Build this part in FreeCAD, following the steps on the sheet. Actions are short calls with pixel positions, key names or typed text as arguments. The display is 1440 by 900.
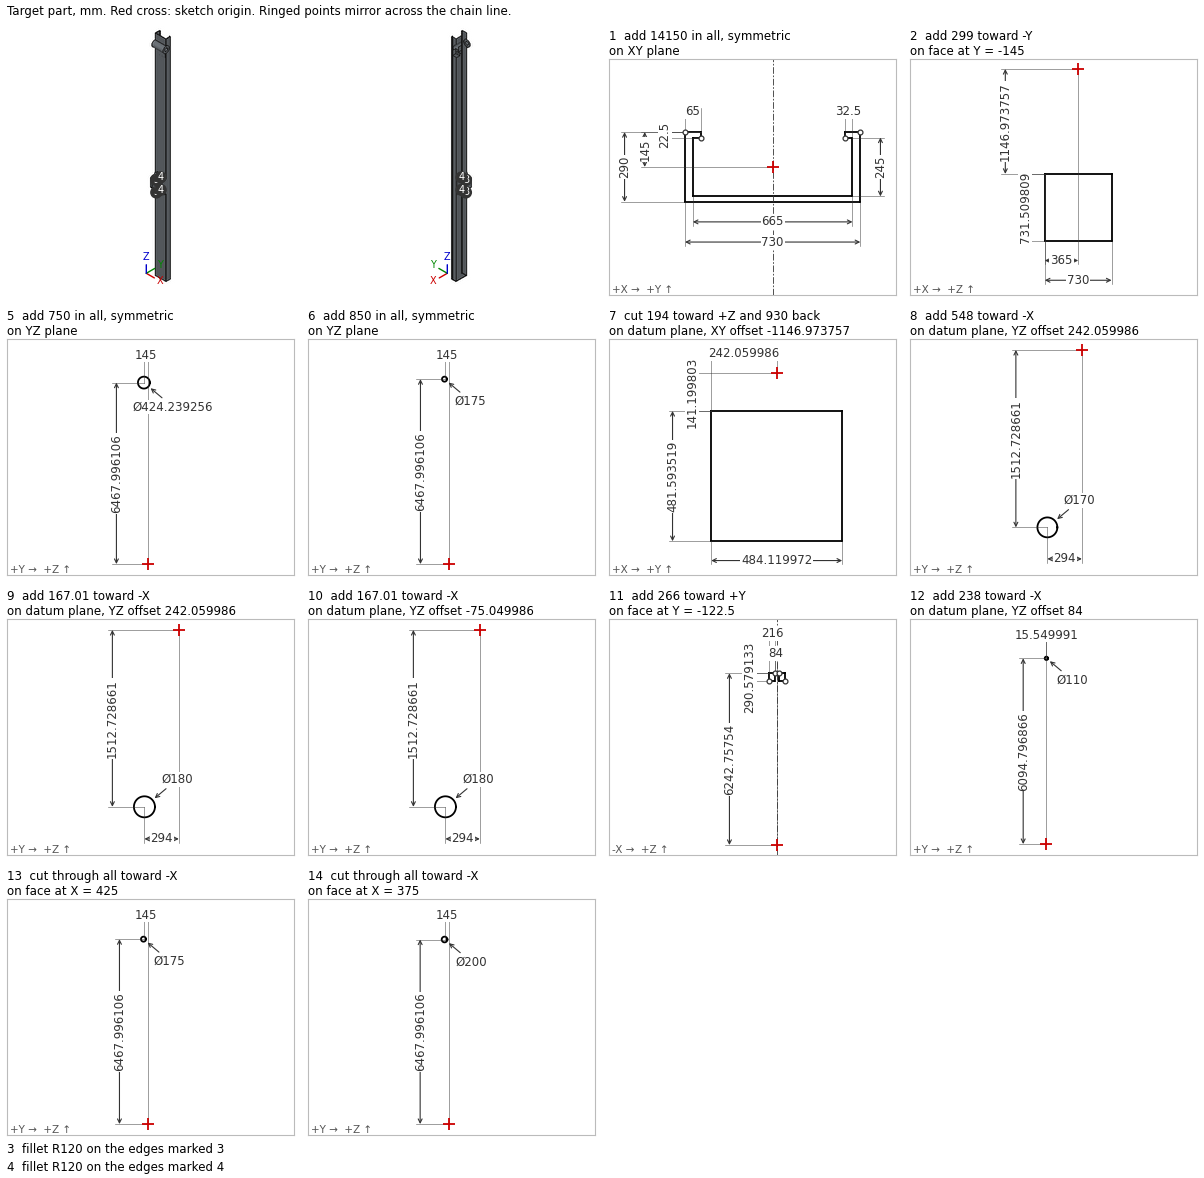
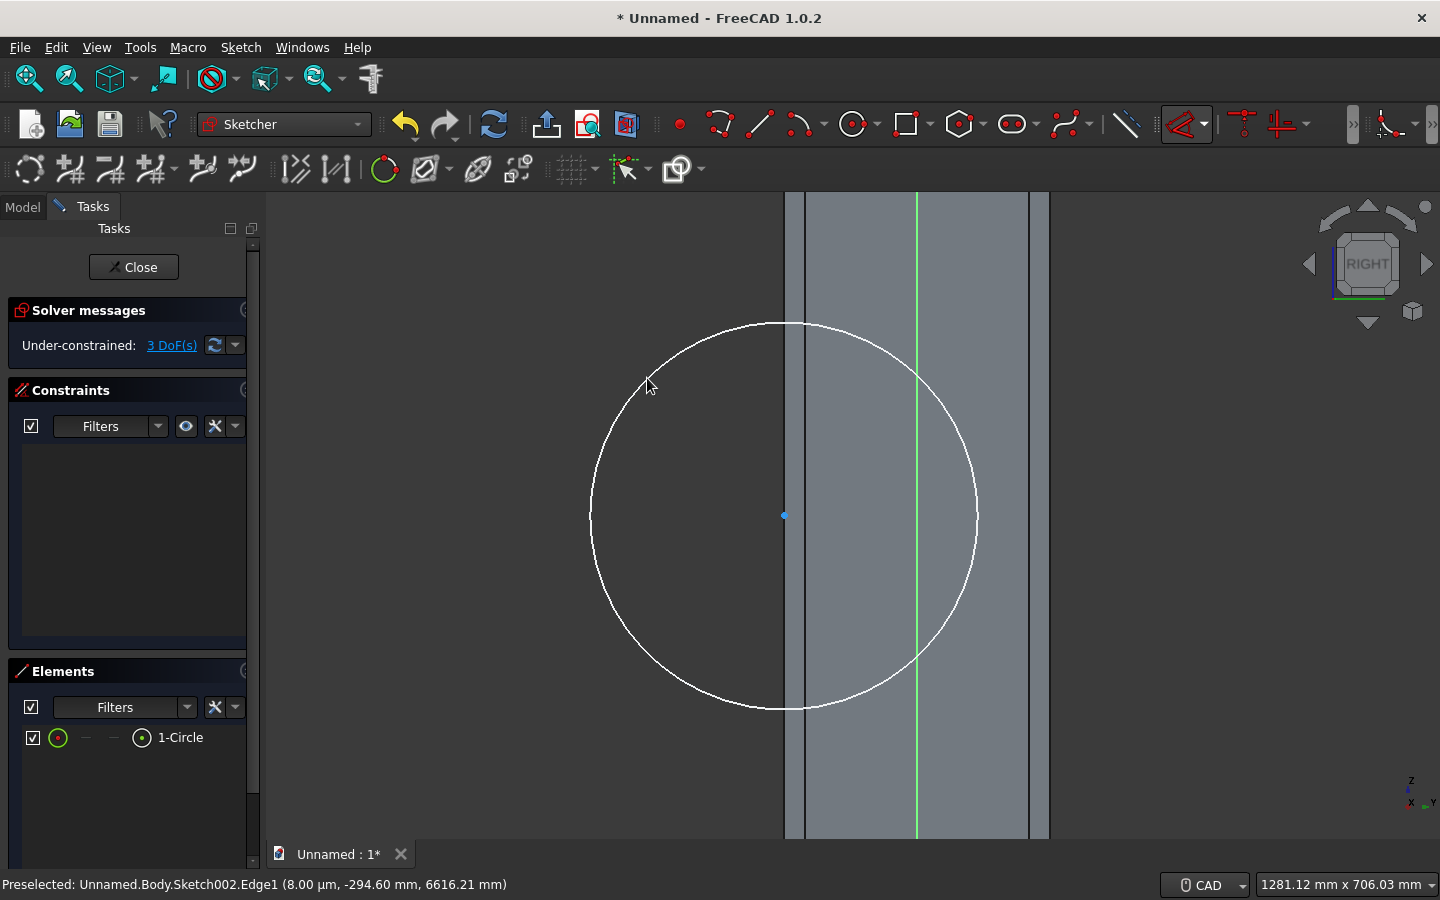
click(921, 379)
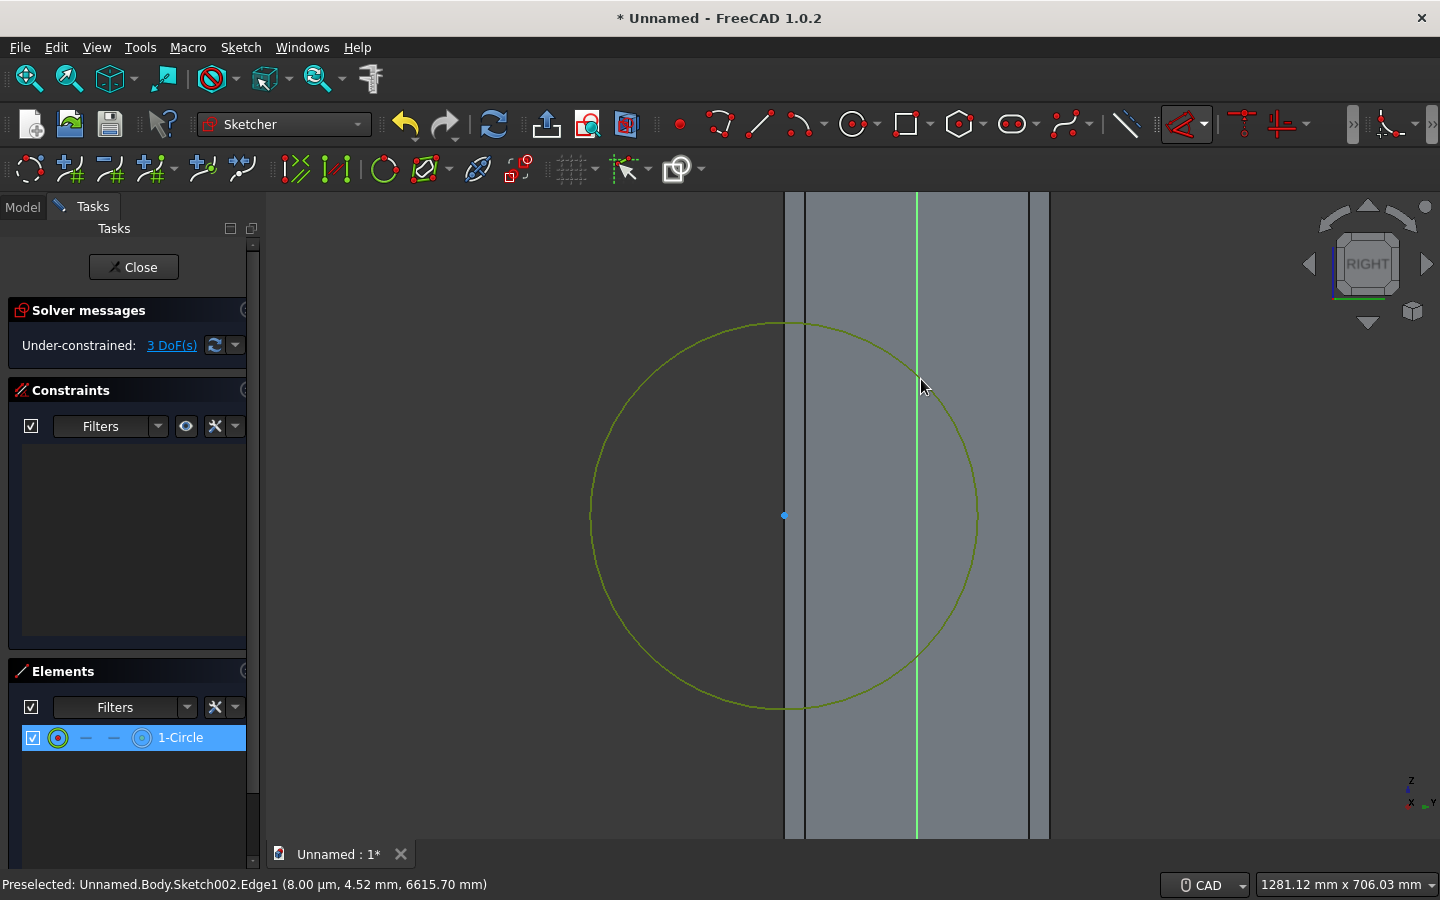
key(k)
key(o)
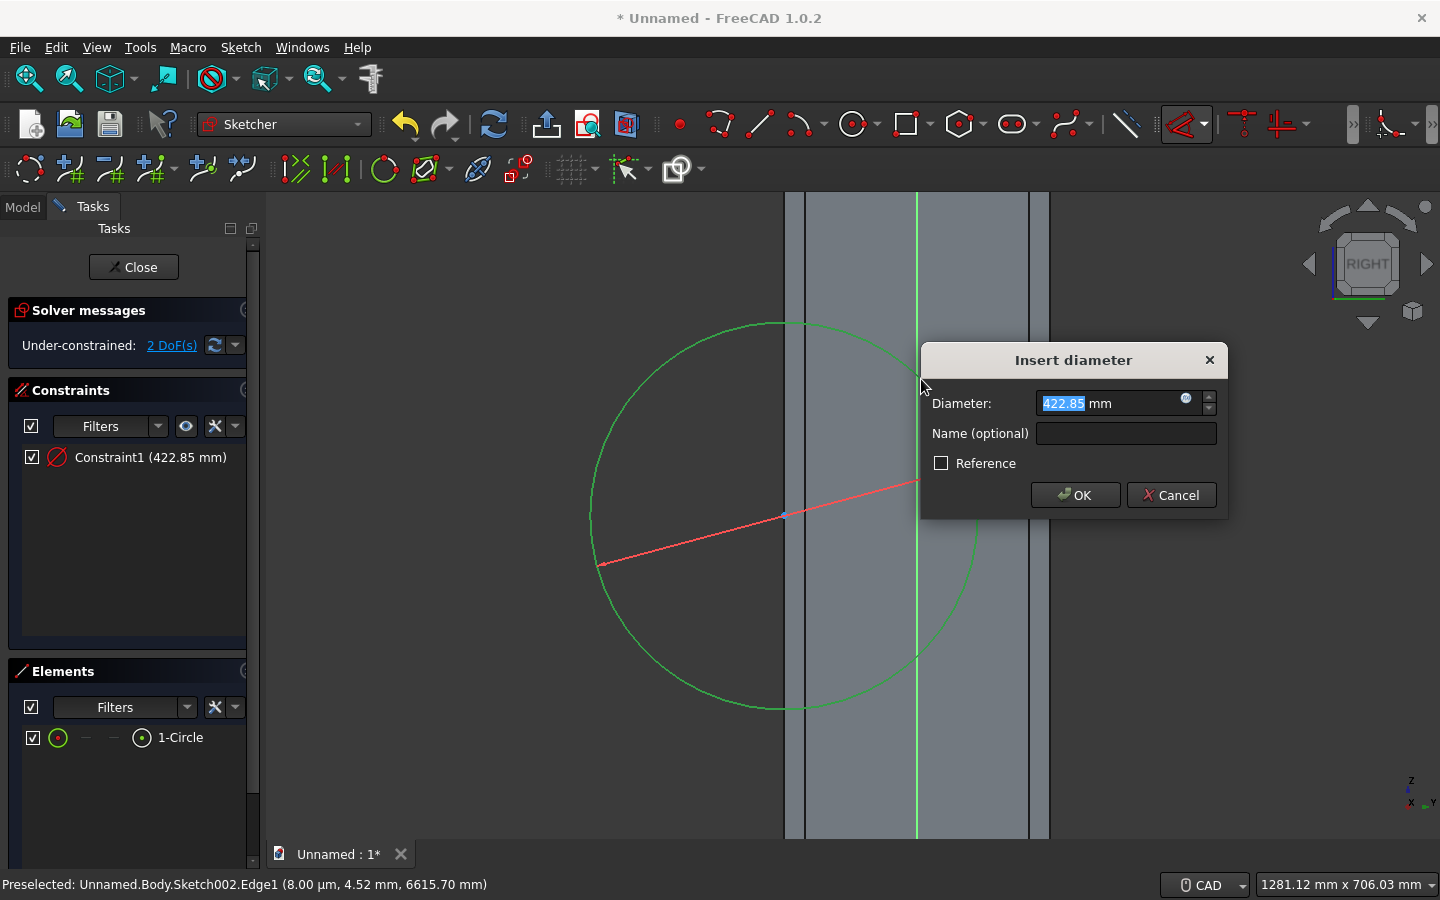
text(424.239256)
key(Return)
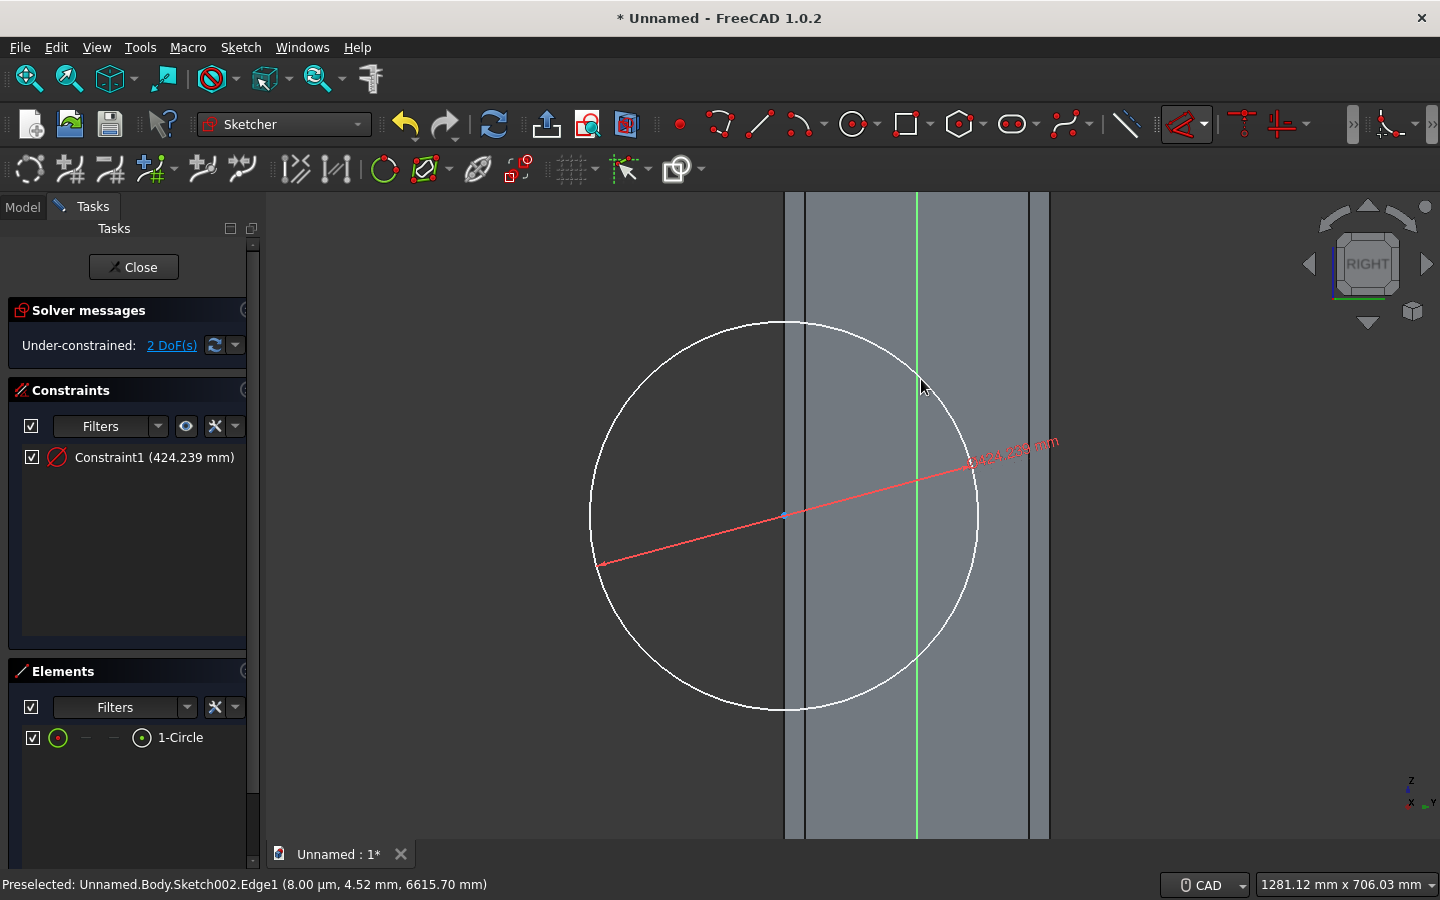
click(784, 516)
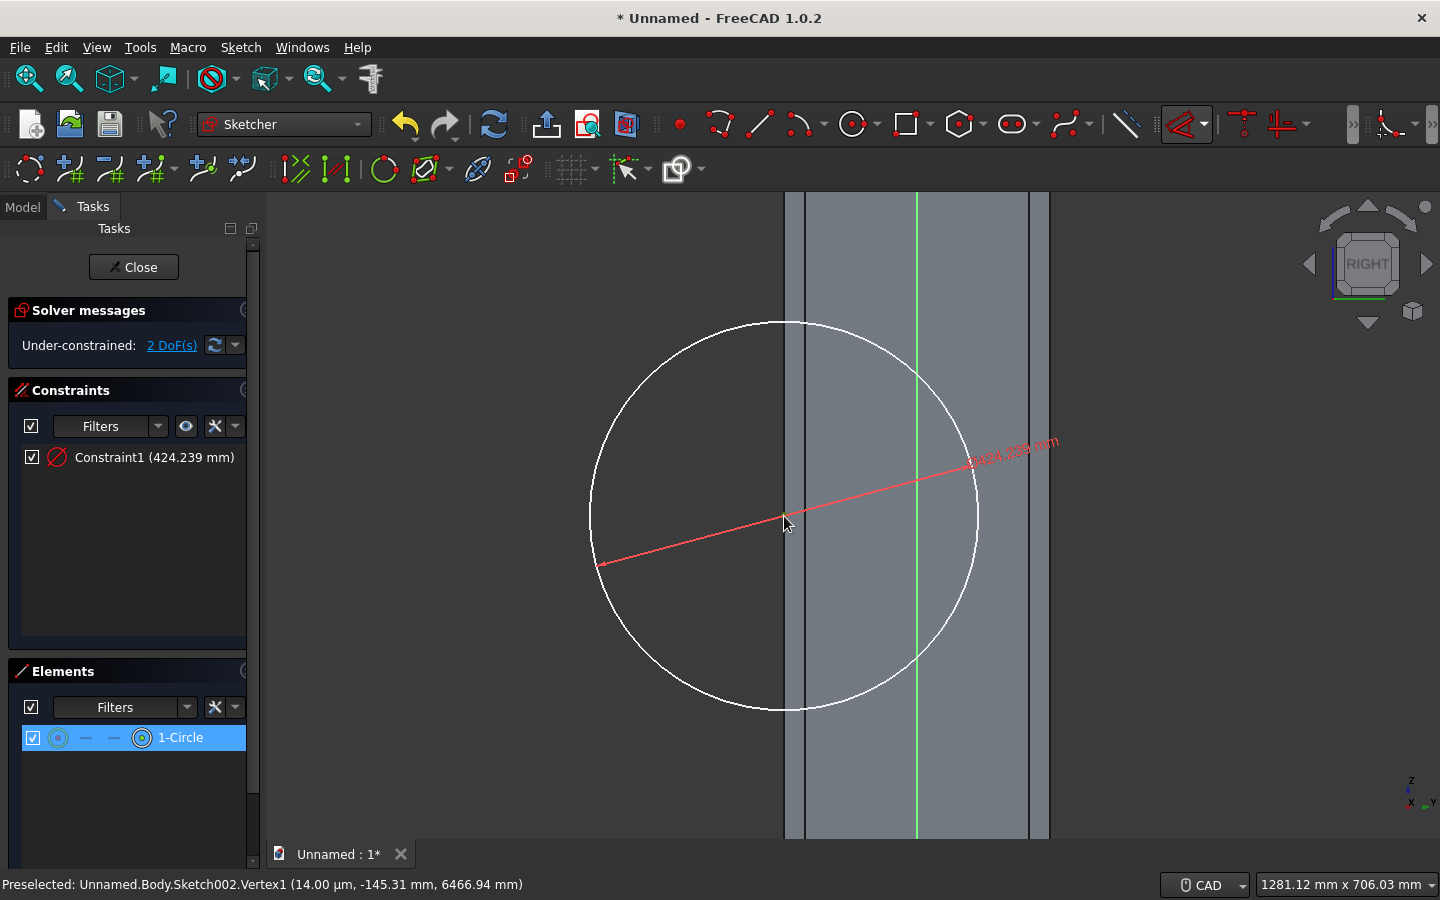
key(l)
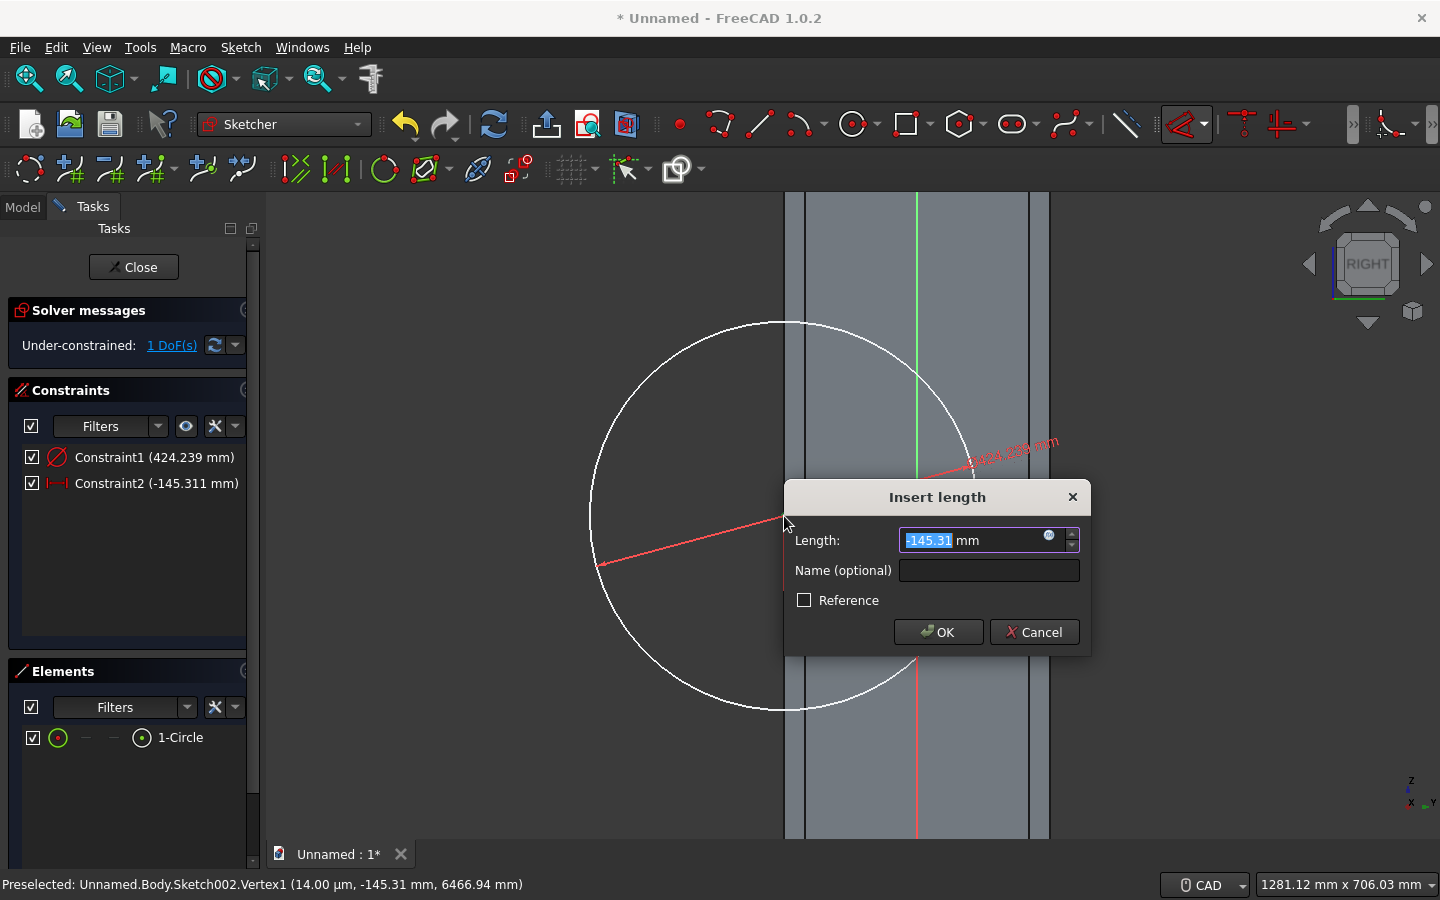
text(-145)
key(Return)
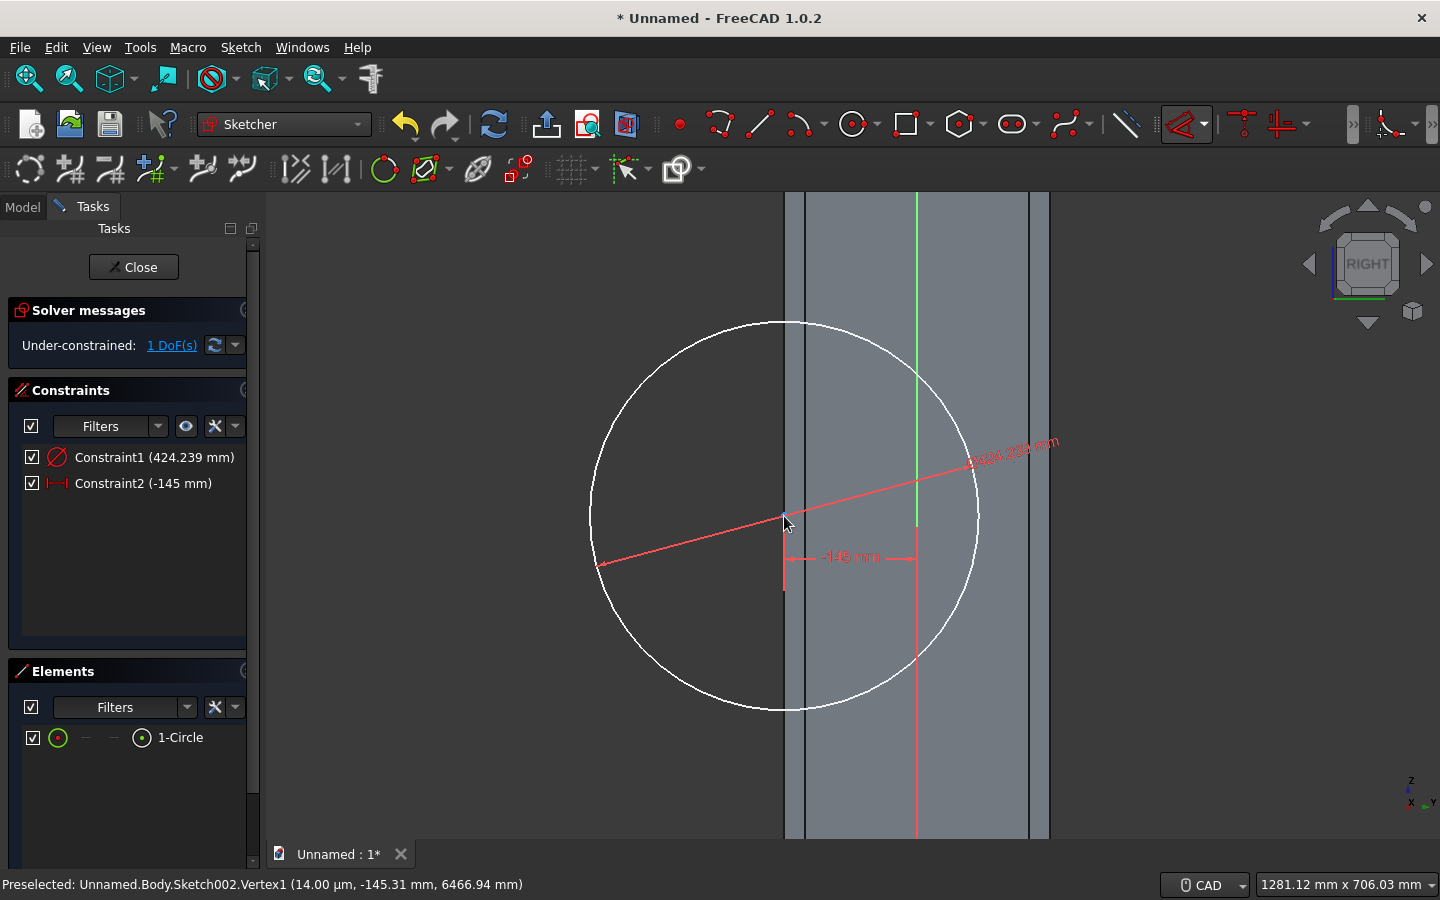
click(784, 516)